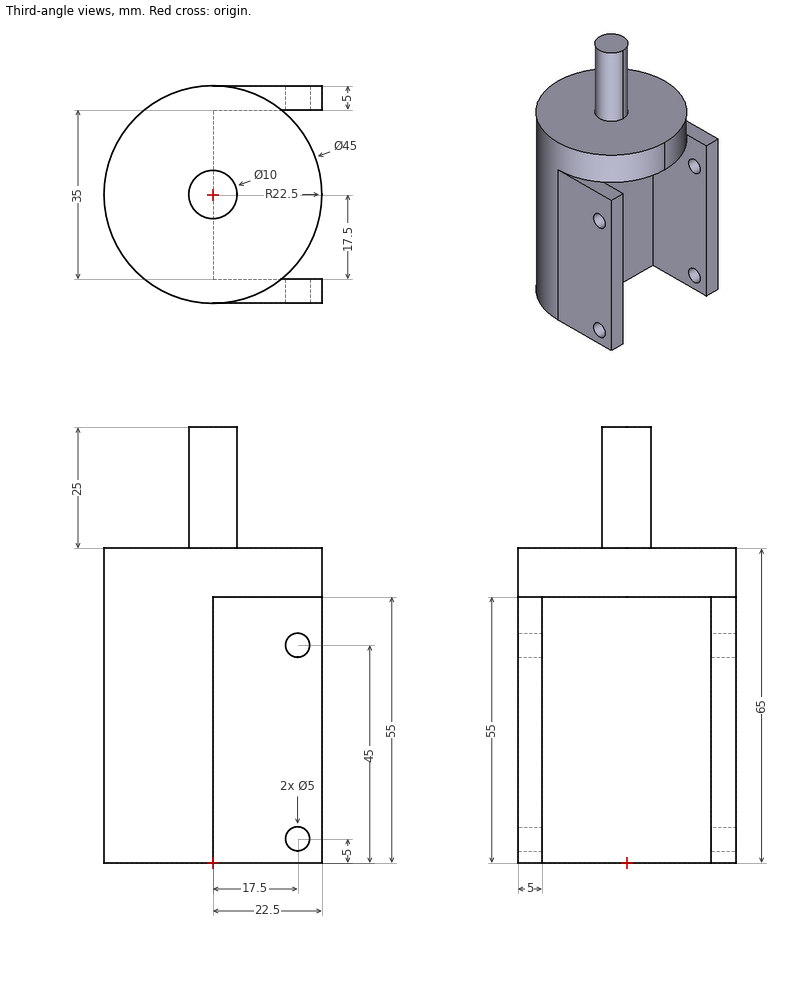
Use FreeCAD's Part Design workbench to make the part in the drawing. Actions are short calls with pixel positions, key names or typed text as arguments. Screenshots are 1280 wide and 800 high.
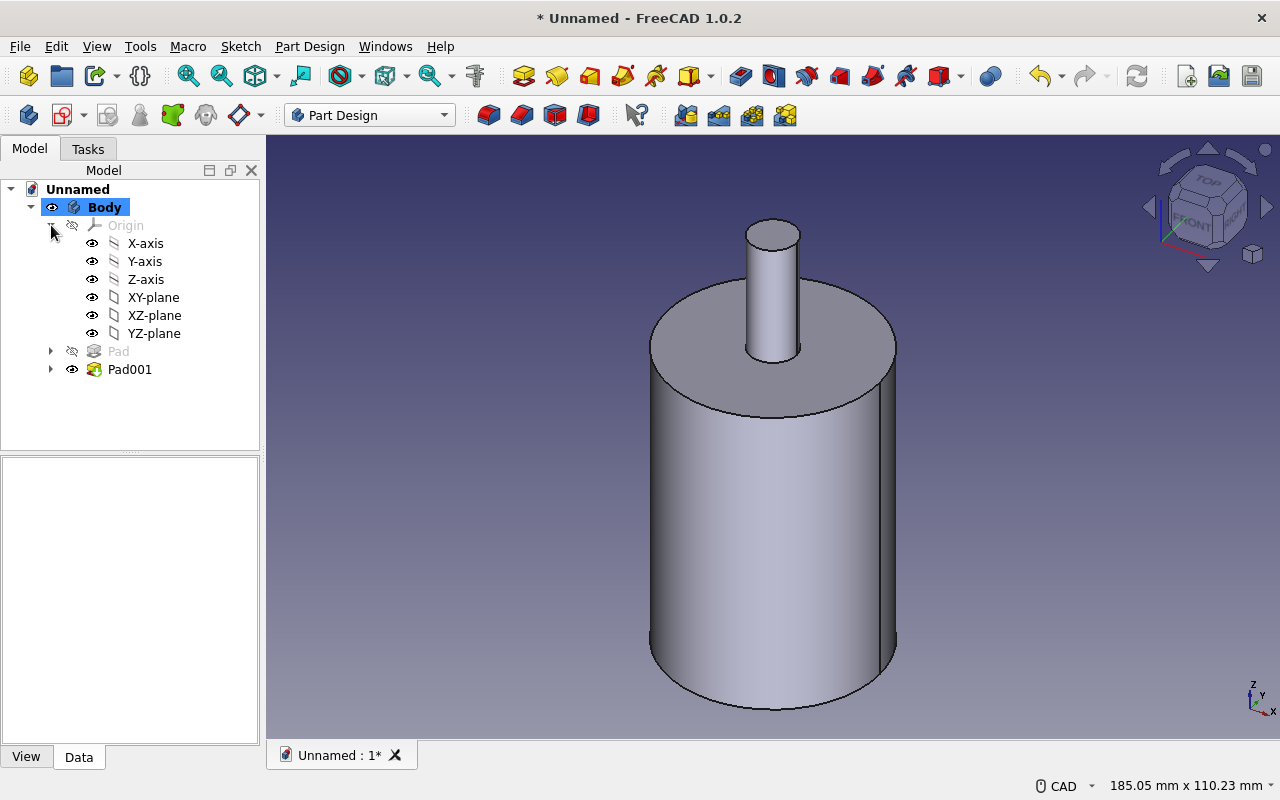
click(137, 315)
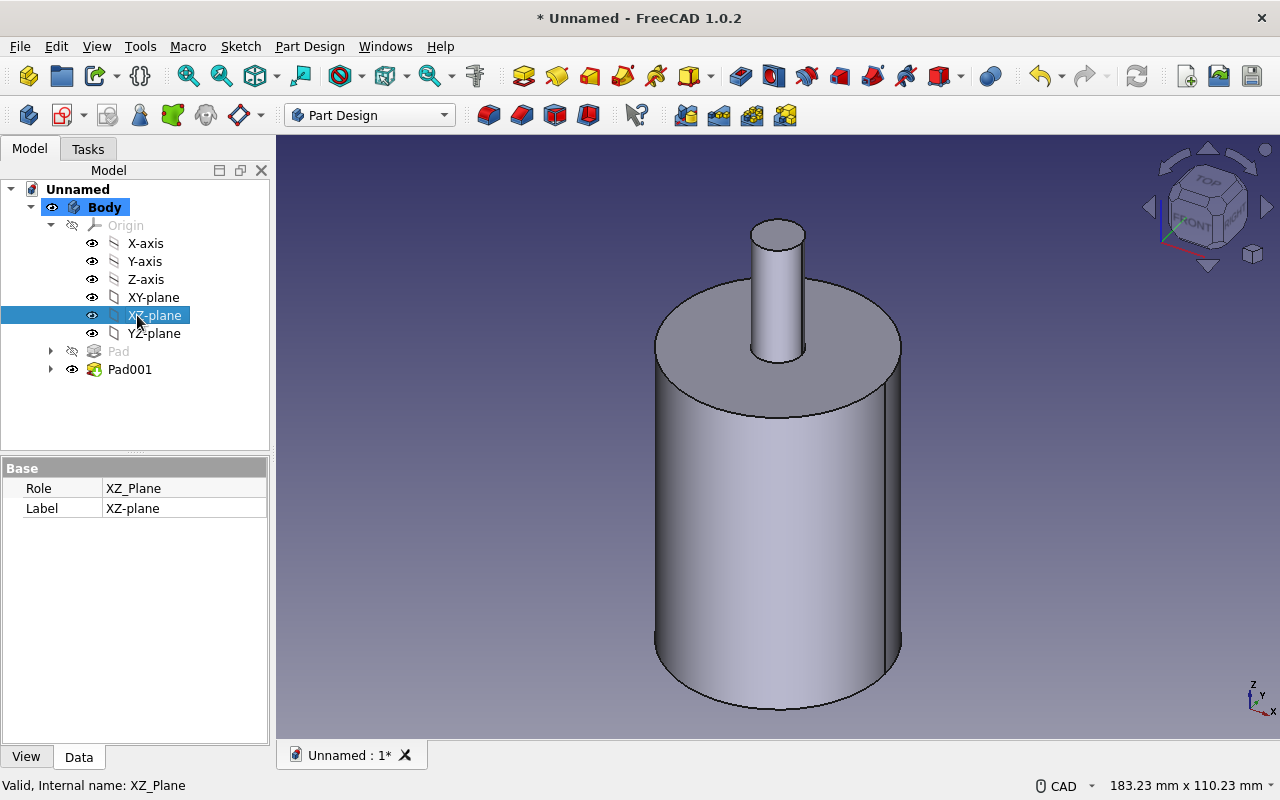
click(238, 116)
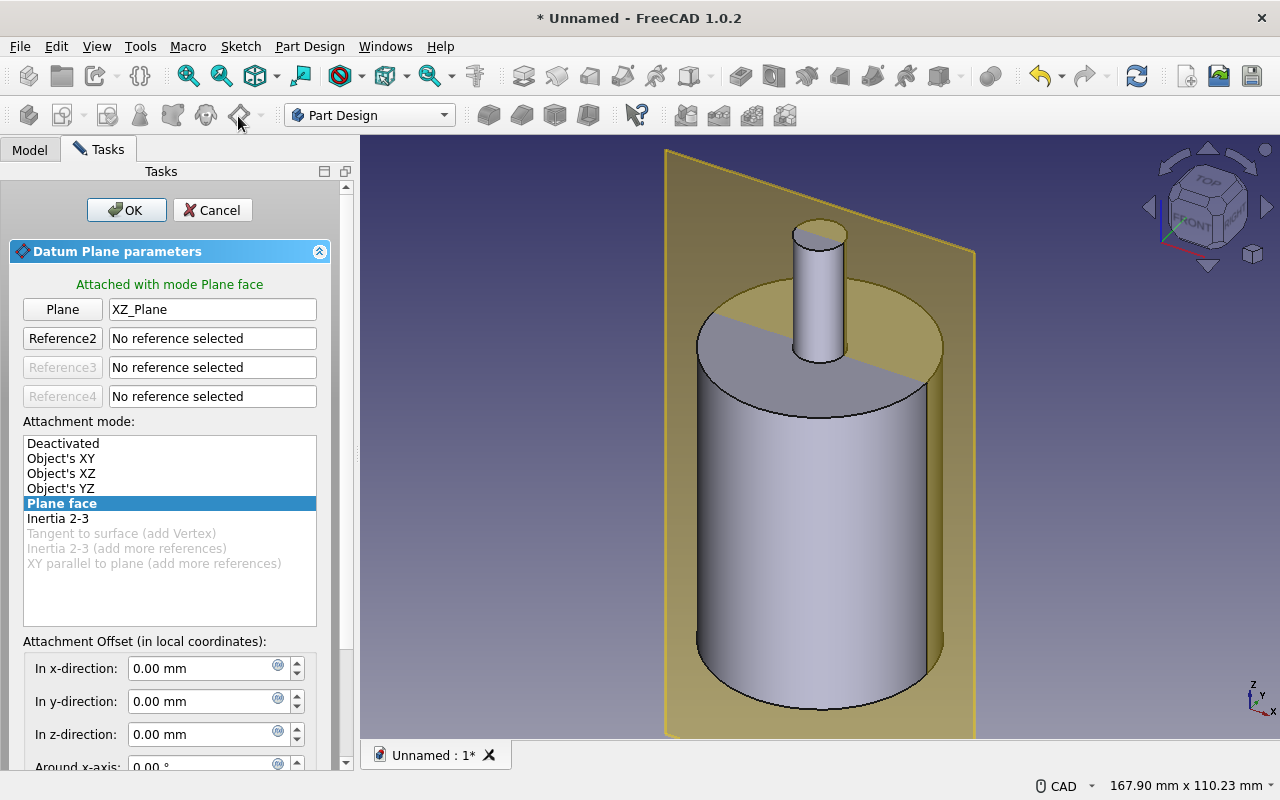
triple_click(210, 734)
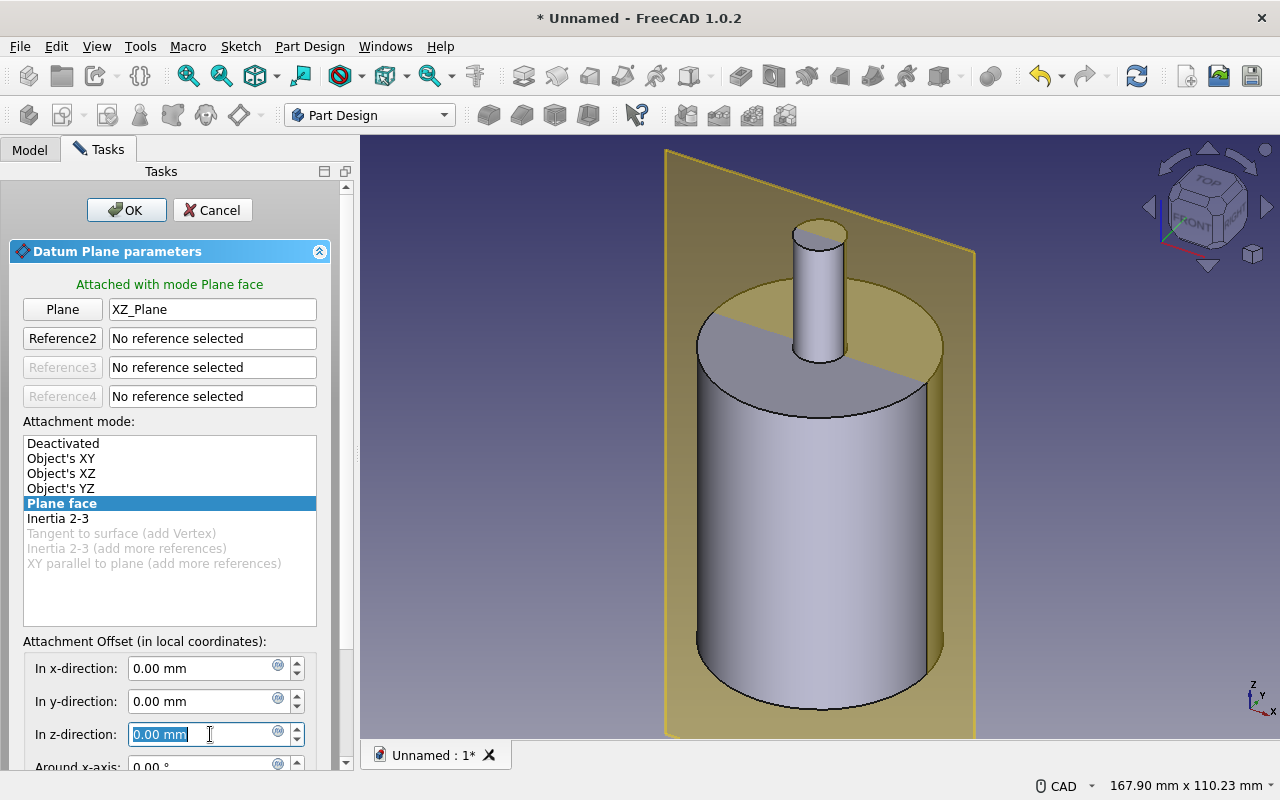
text(-22.5)
key(Tab)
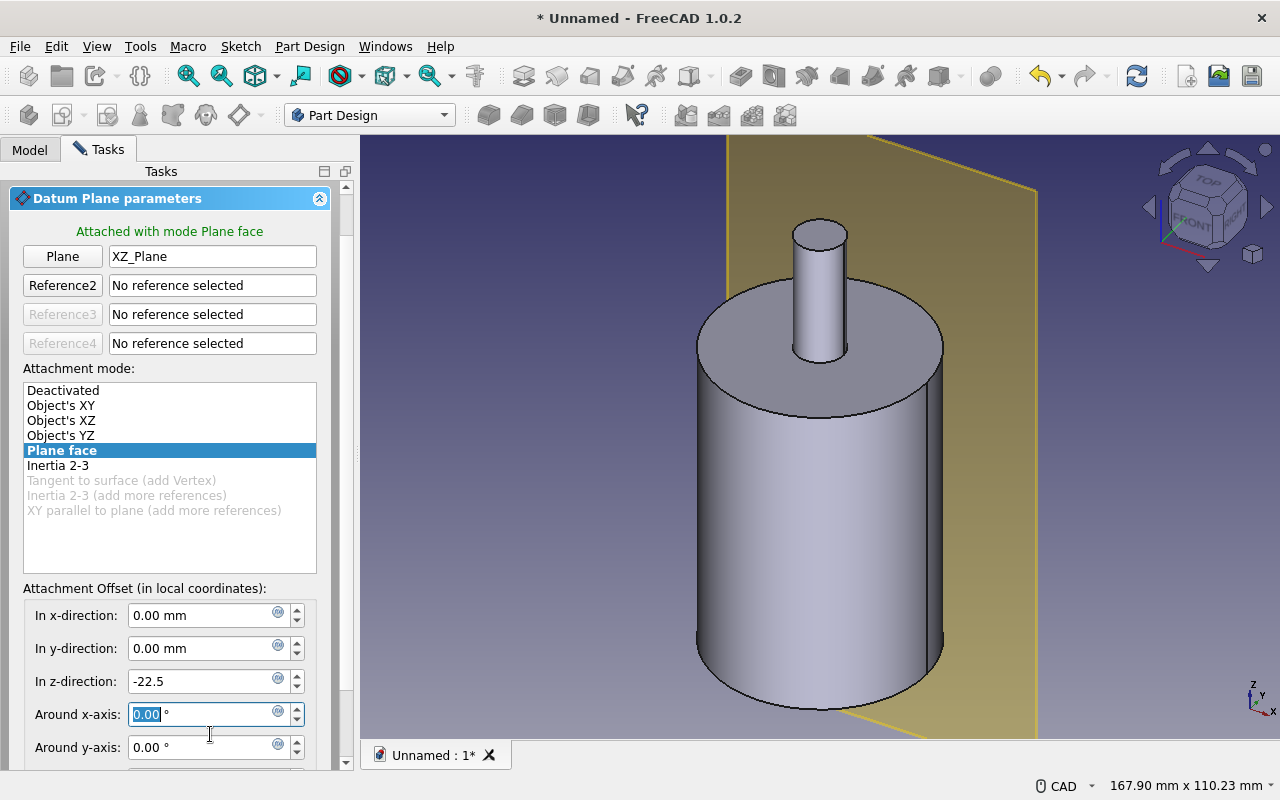
scroll(346, 476, up, 2)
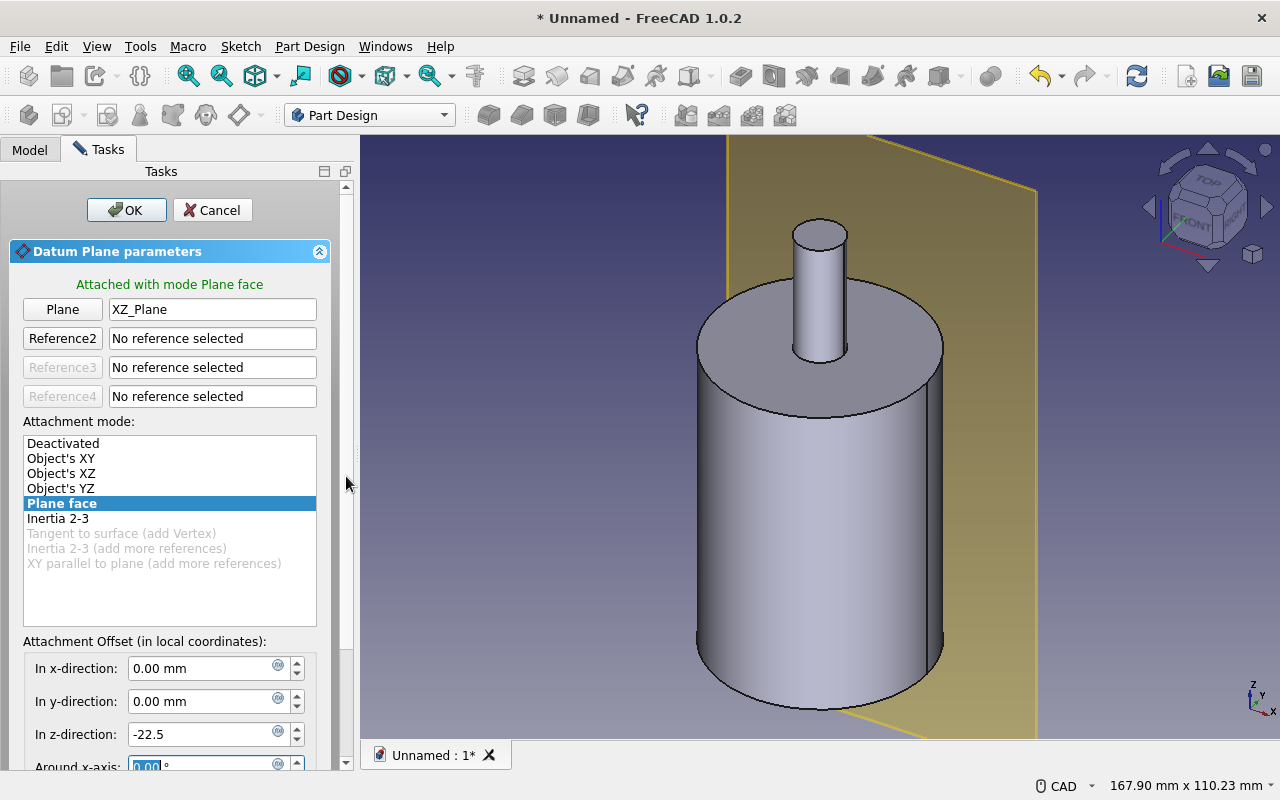
click(127, 210)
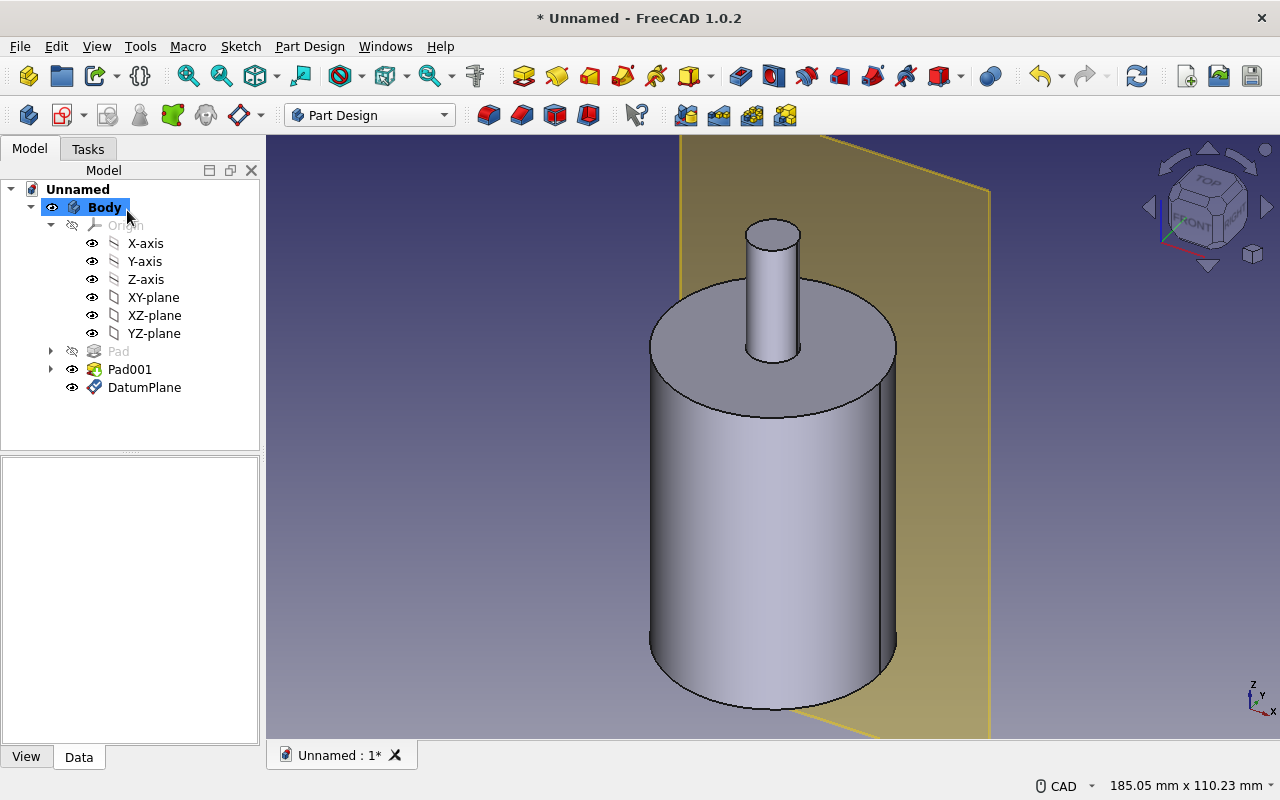
click(117, 387)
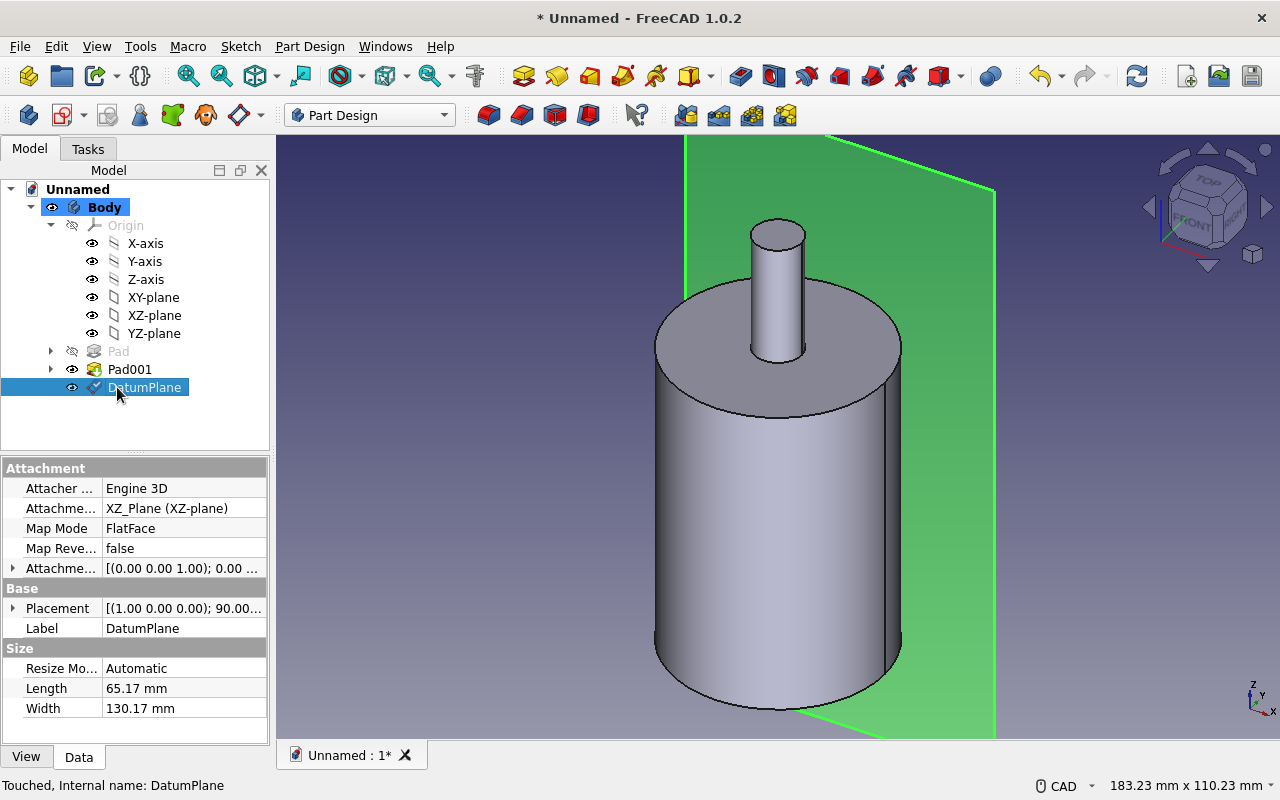
click(62, 116)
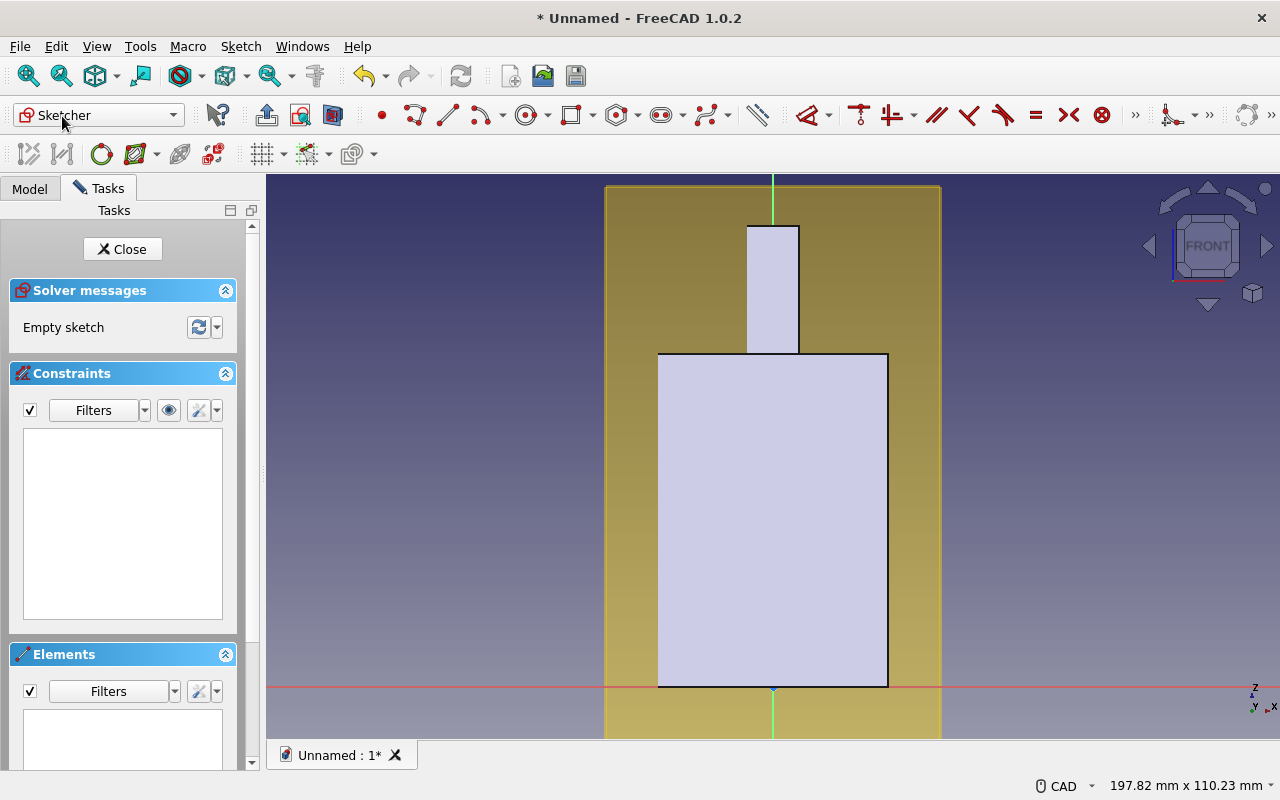
click(333, 116)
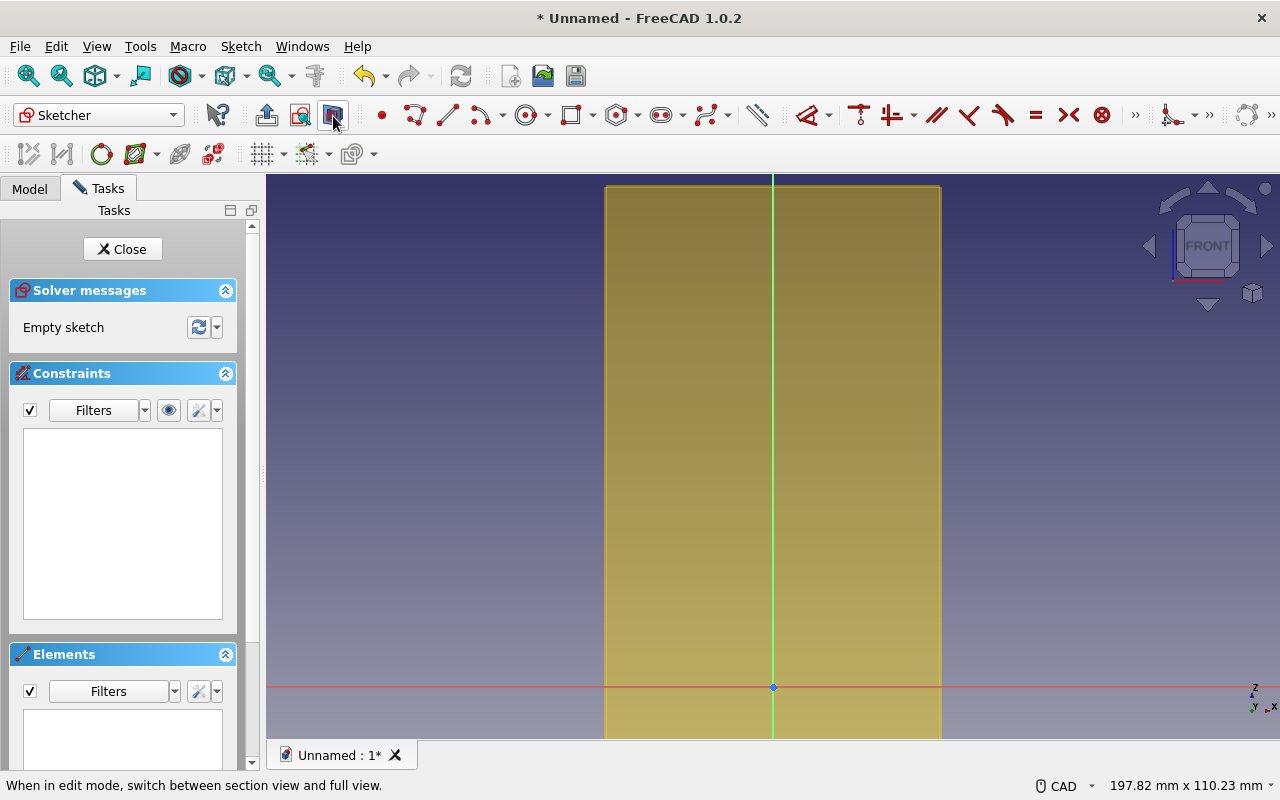
scroll(1115, 711, up, 1)